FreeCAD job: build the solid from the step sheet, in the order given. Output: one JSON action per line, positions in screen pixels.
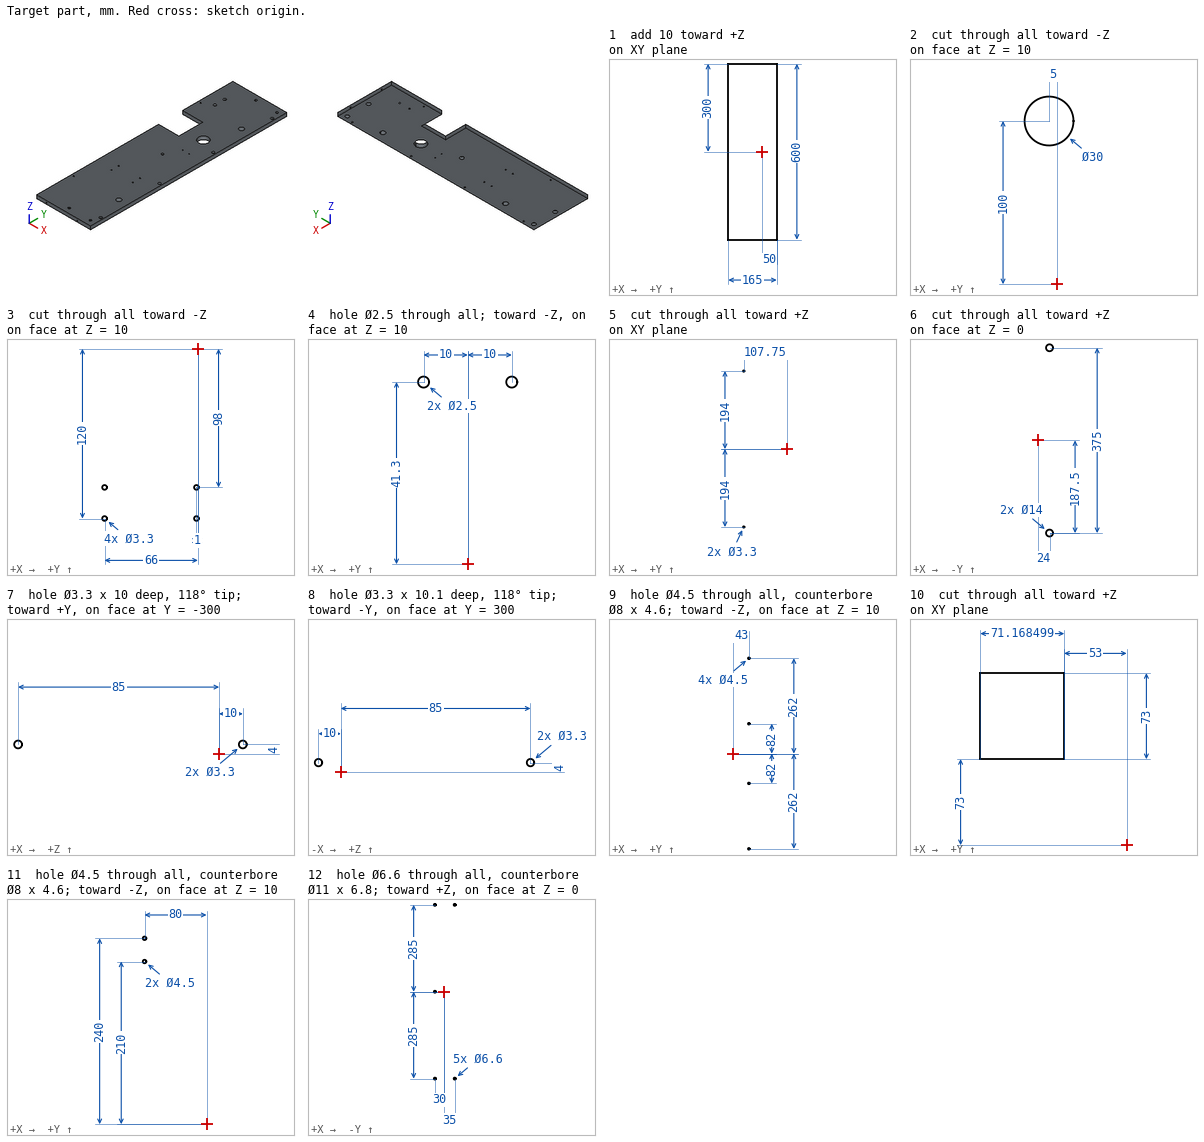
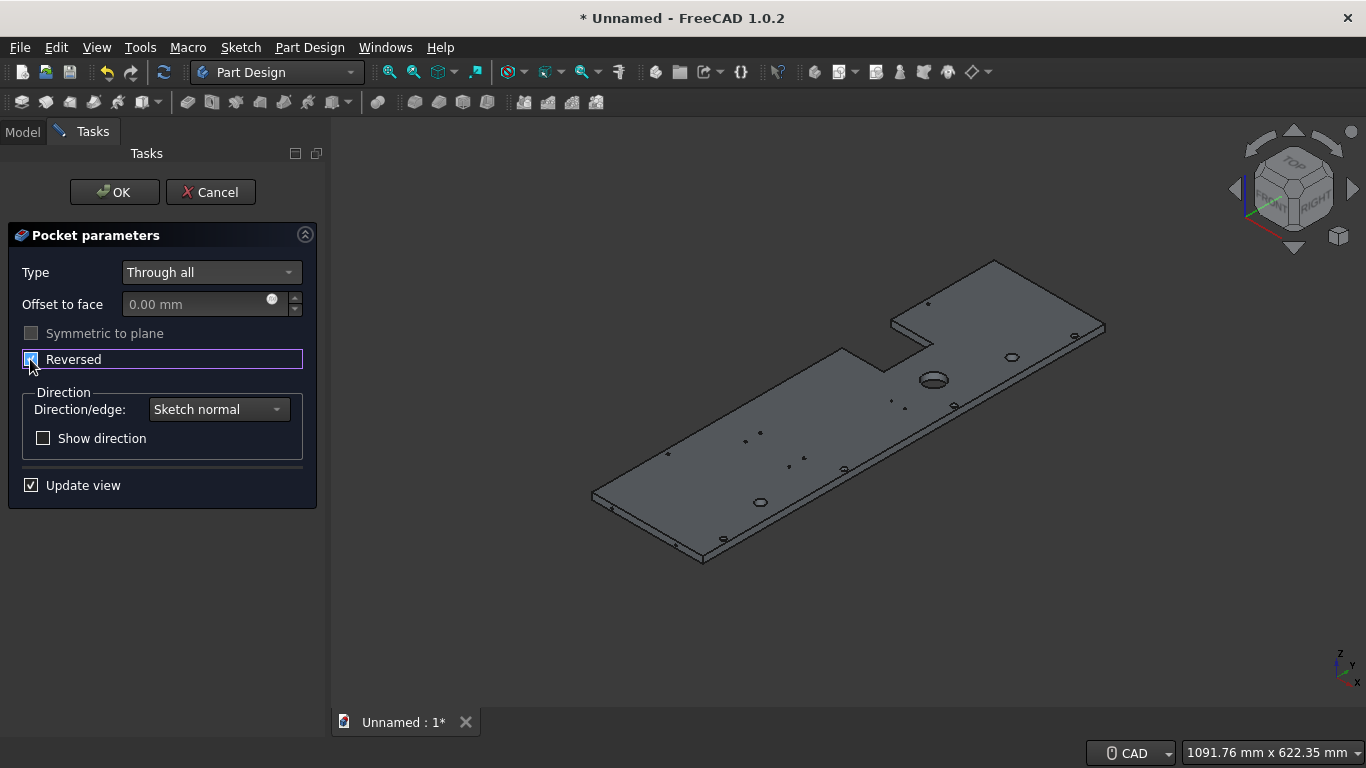
{"action": "left_click", "coordinate": [115, 192]}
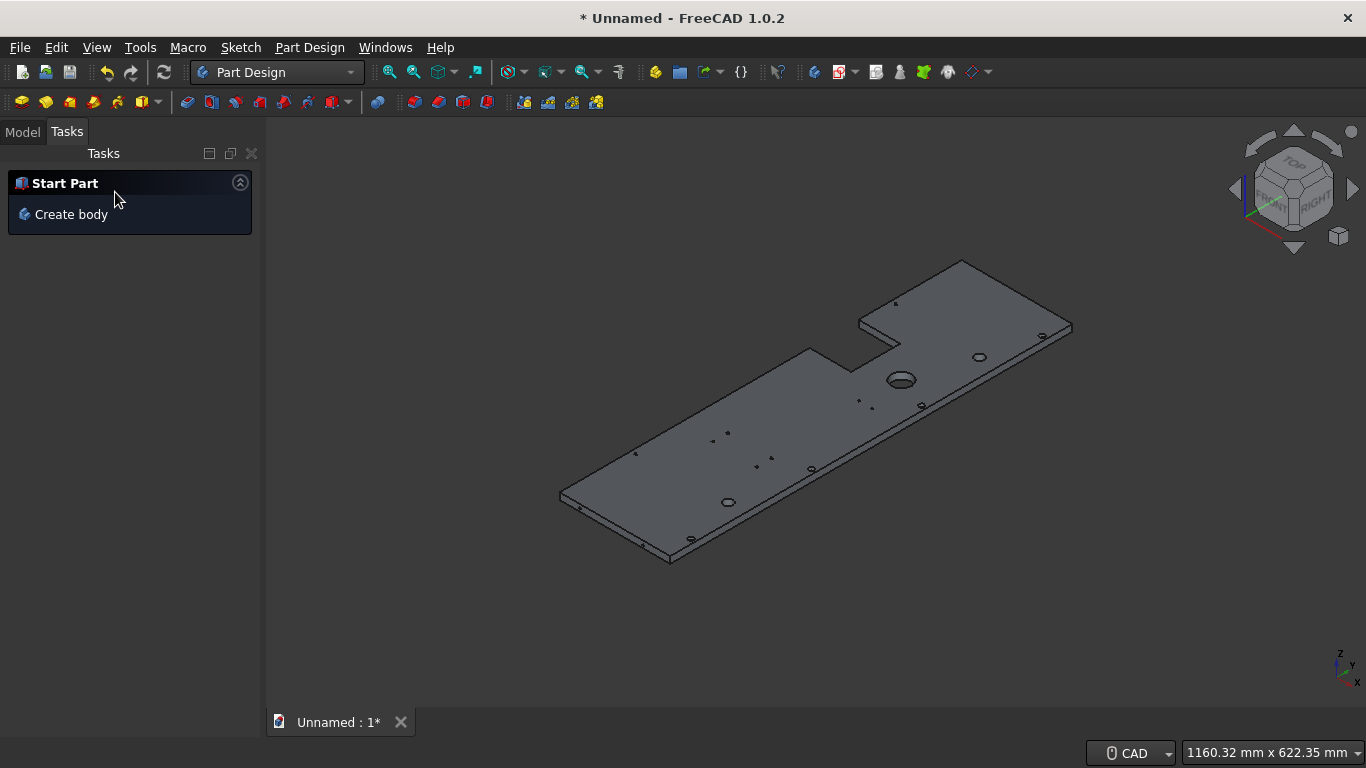
{"action": "left_click", "coordinate": [800, 398]}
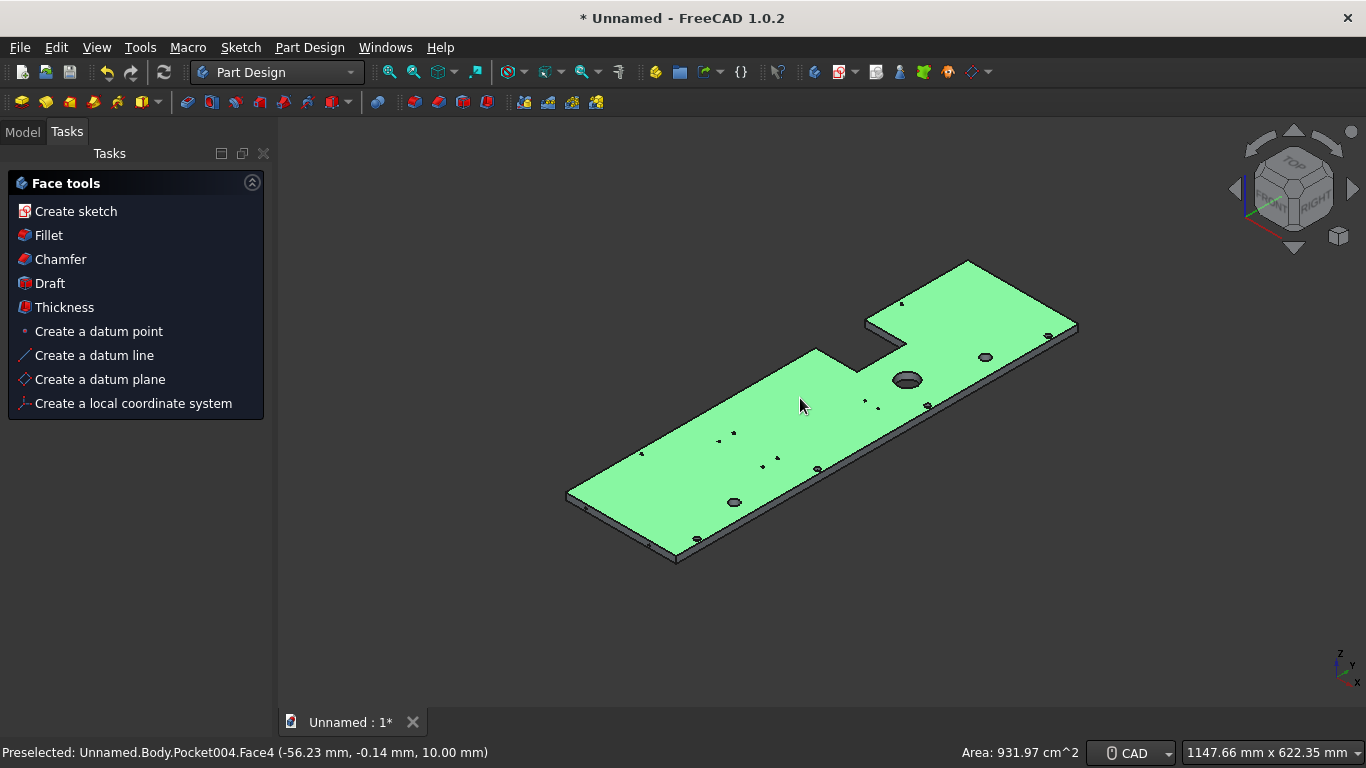
{"action": "left_click", "coordinate": [840, 72]}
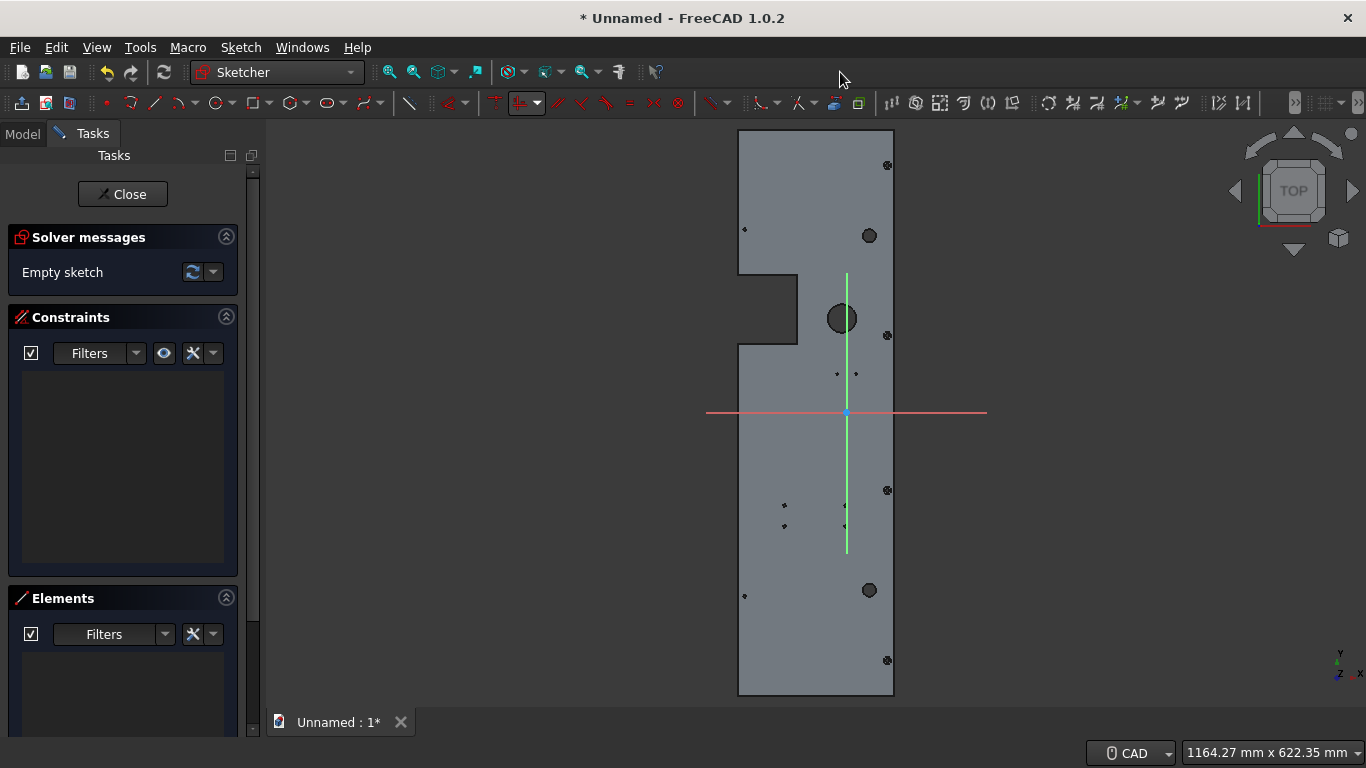
{"action": "scroll", "coordinate": [773, 179], "scroll_direction": "up", "scroll_amount": 12}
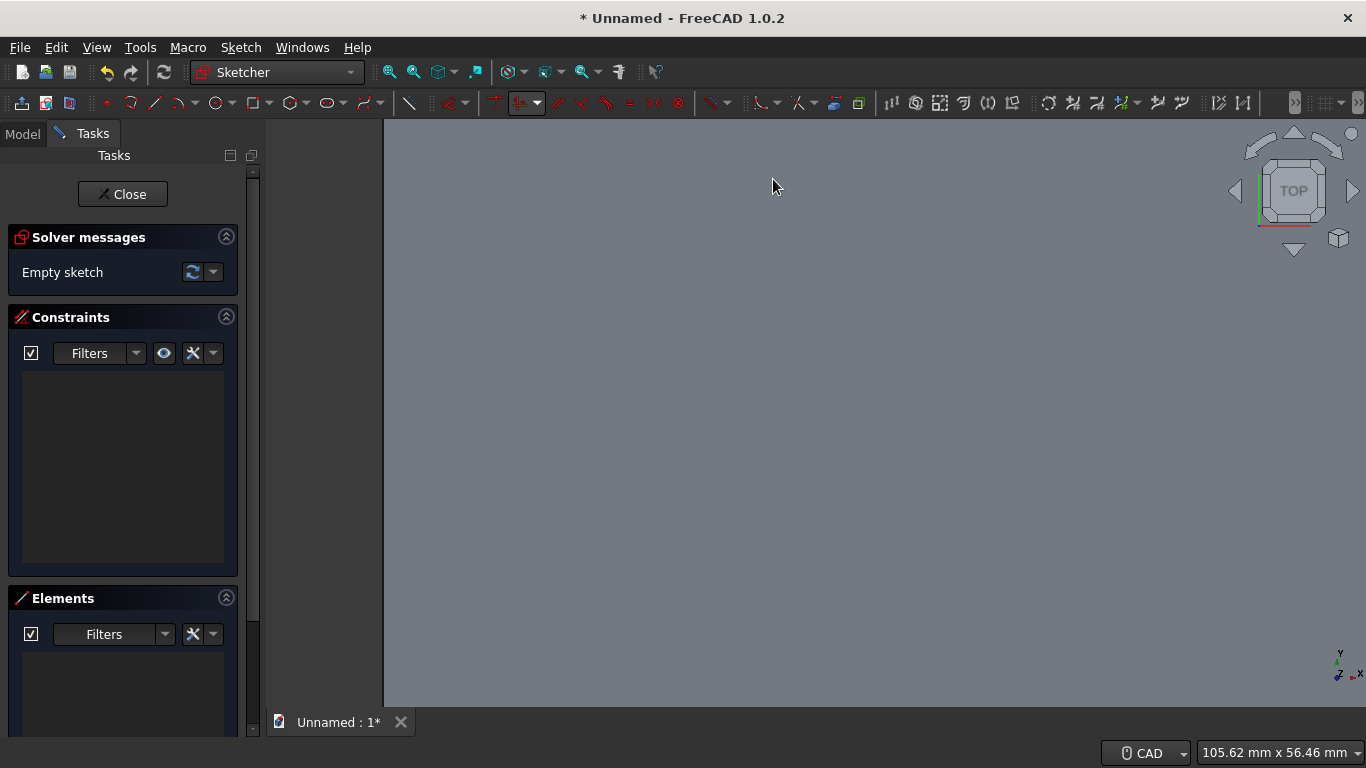
{"action": "left_click", "coordinate": [216, 104]}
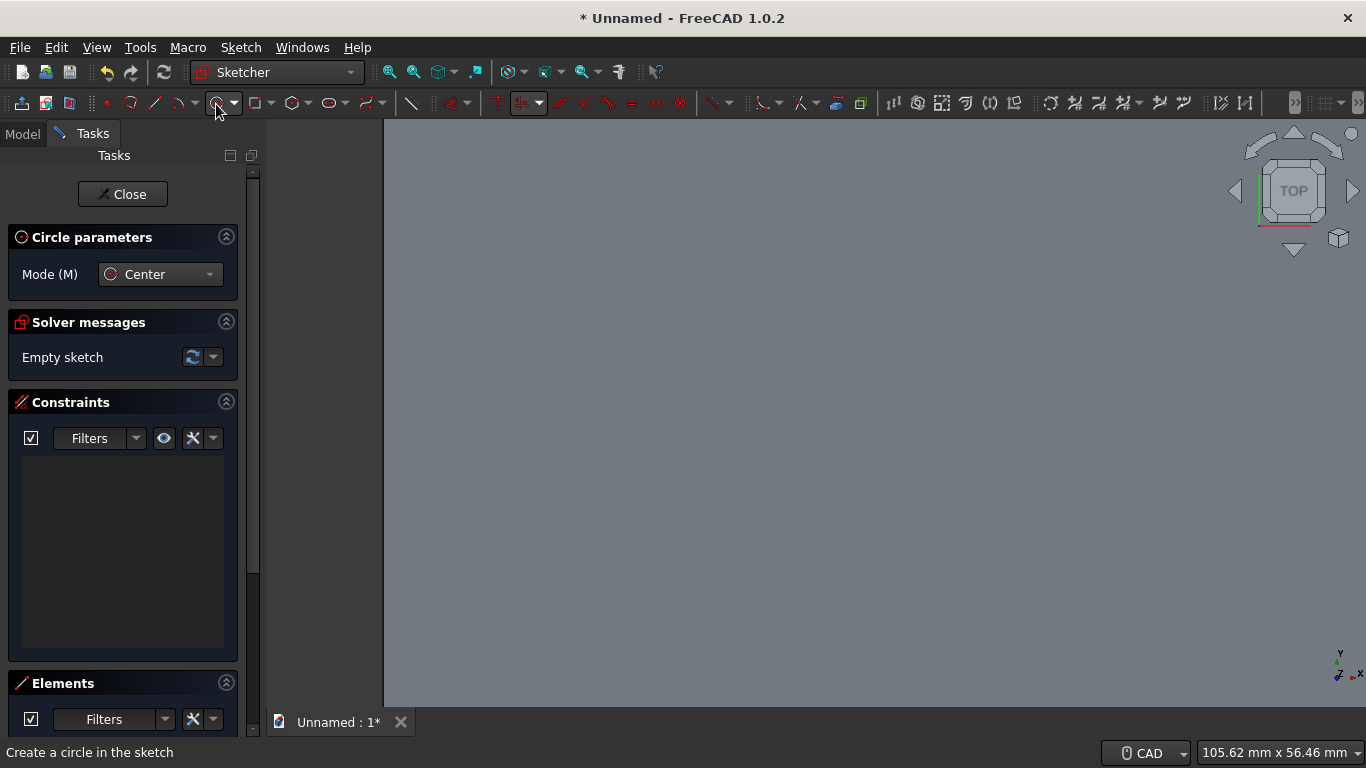
{"action": "left_click", "coordinate": [748, 258]}
{"action": "mouse_move", "coordinate": [764, 241]}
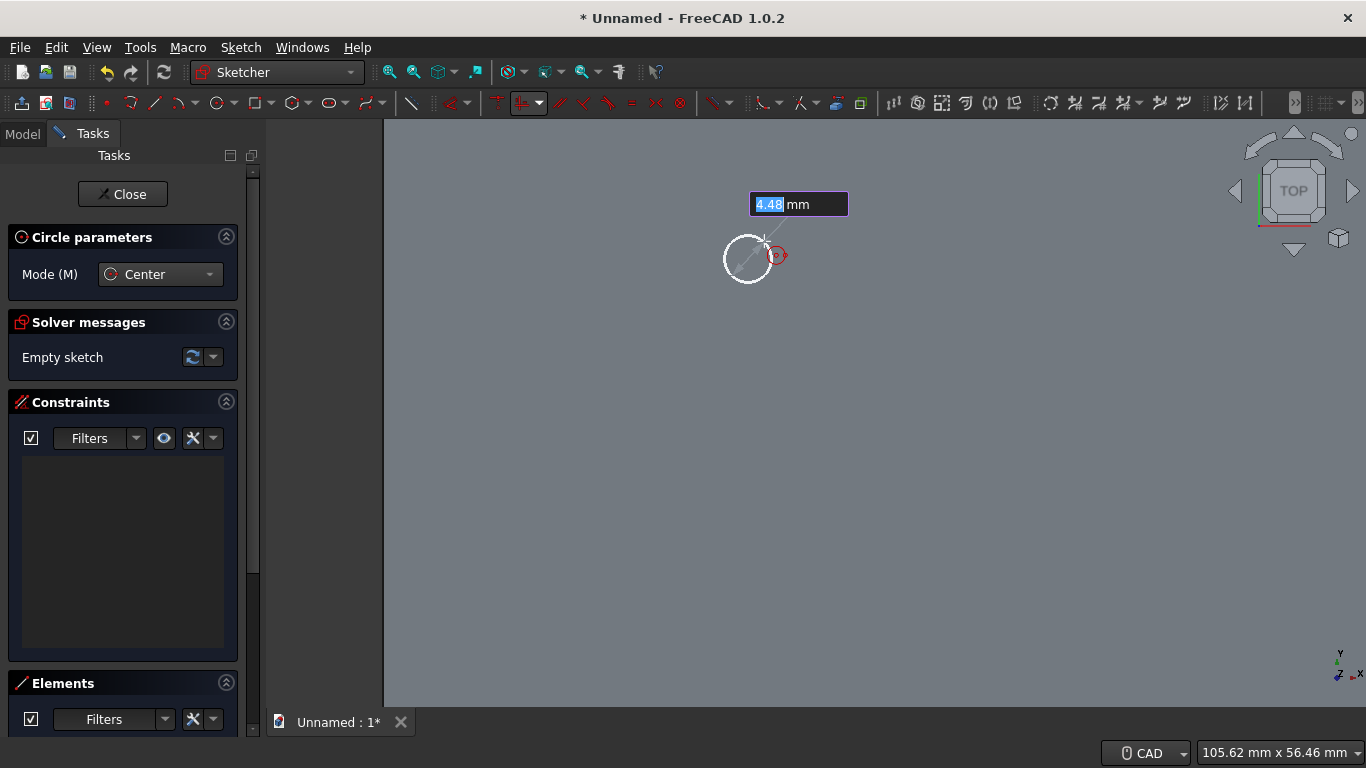
{"action": "type", "text": "4.5"}
{"action": "key", "text": "Return"}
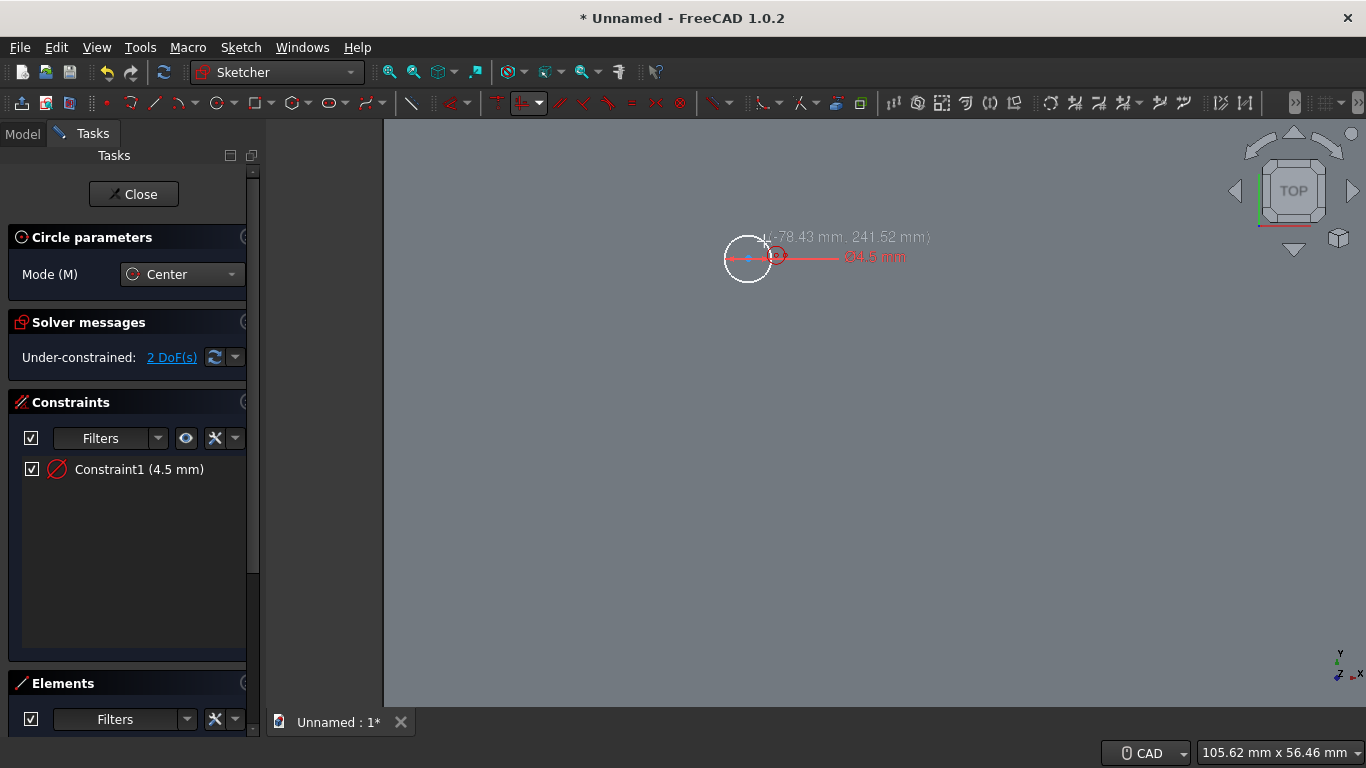
{"action": "left_click", "coordinate": [748, 570]}
{"action": "mouse_move", "coordinate": [764, 554]}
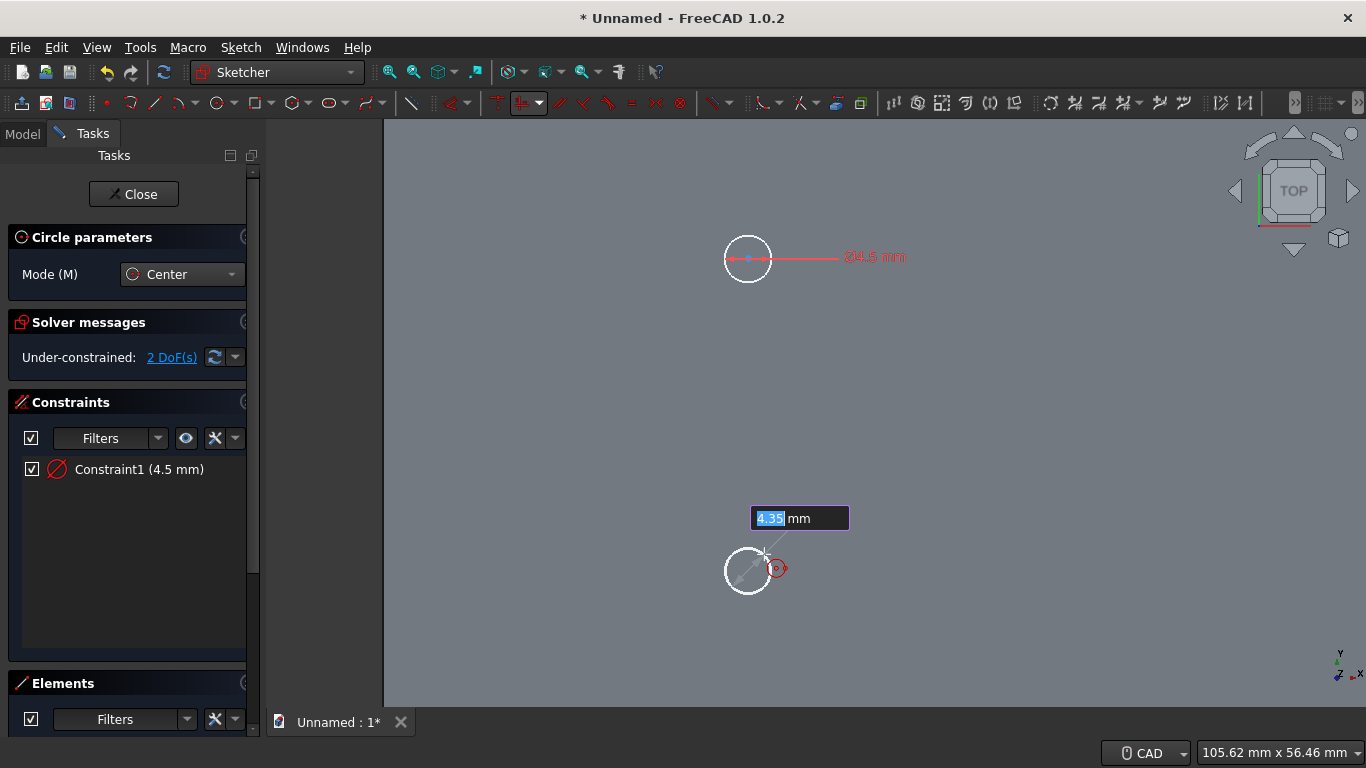
{"action": "type", "text": "4.5"}
{"action": "key", "text": "Return"}
{"action": "key", "text": "Escape"}